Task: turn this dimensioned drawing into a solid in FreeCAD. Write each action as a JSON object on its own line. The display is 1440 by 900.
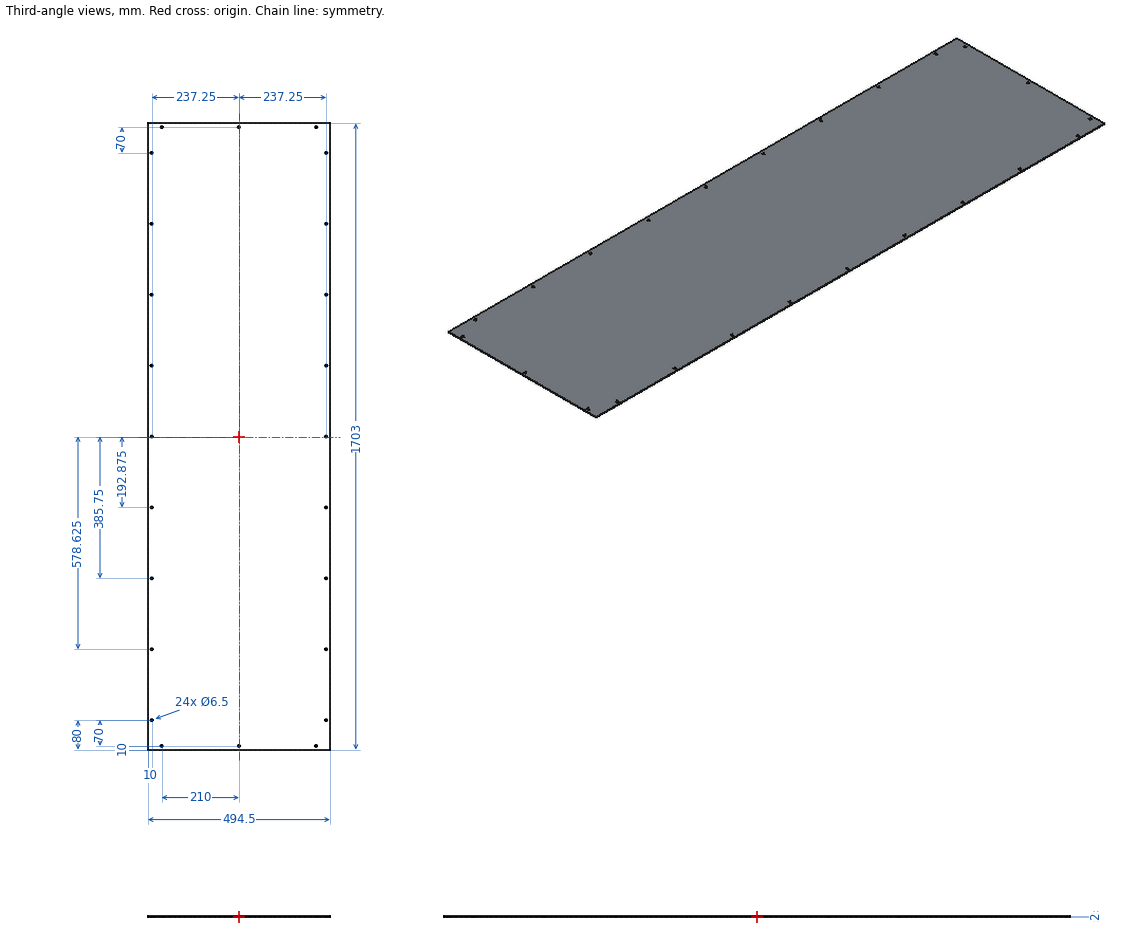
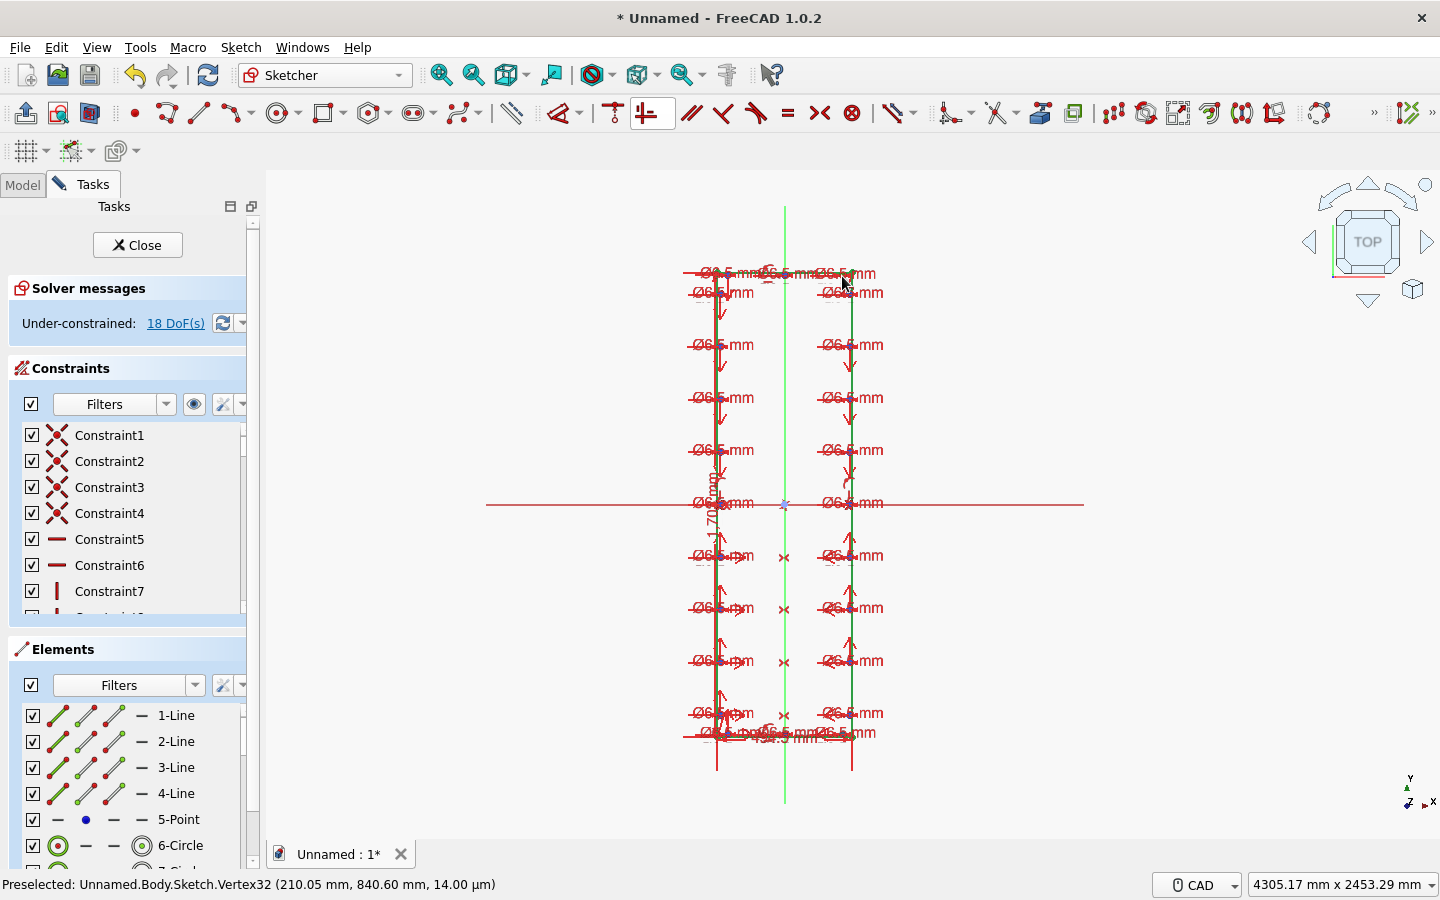
{"action": "left_click", "coordinate": [504, 505]}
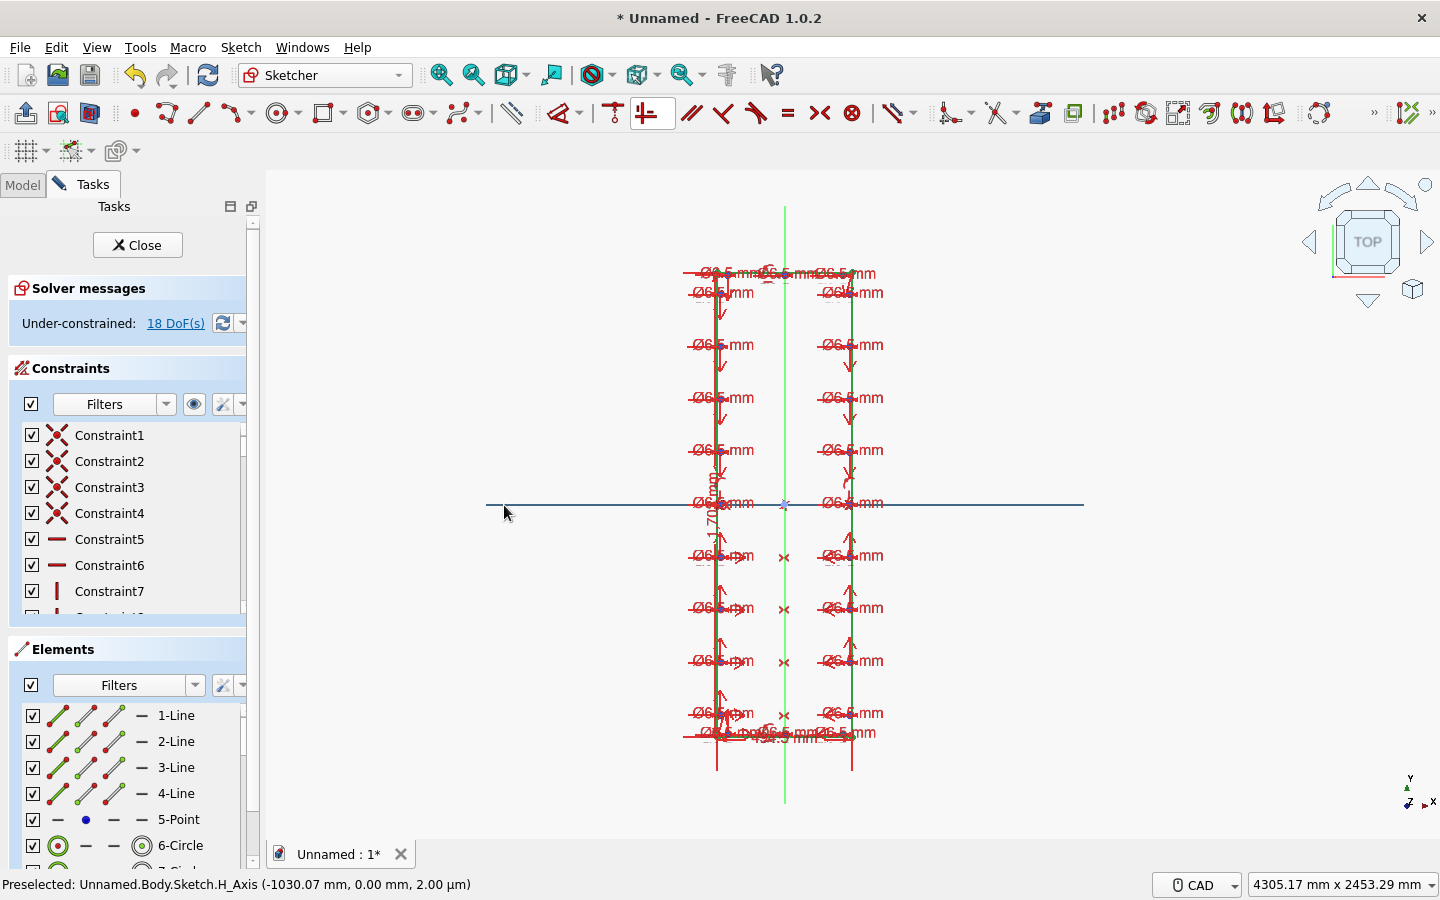
{"action": "left_click", "coordinate": [820, 114]}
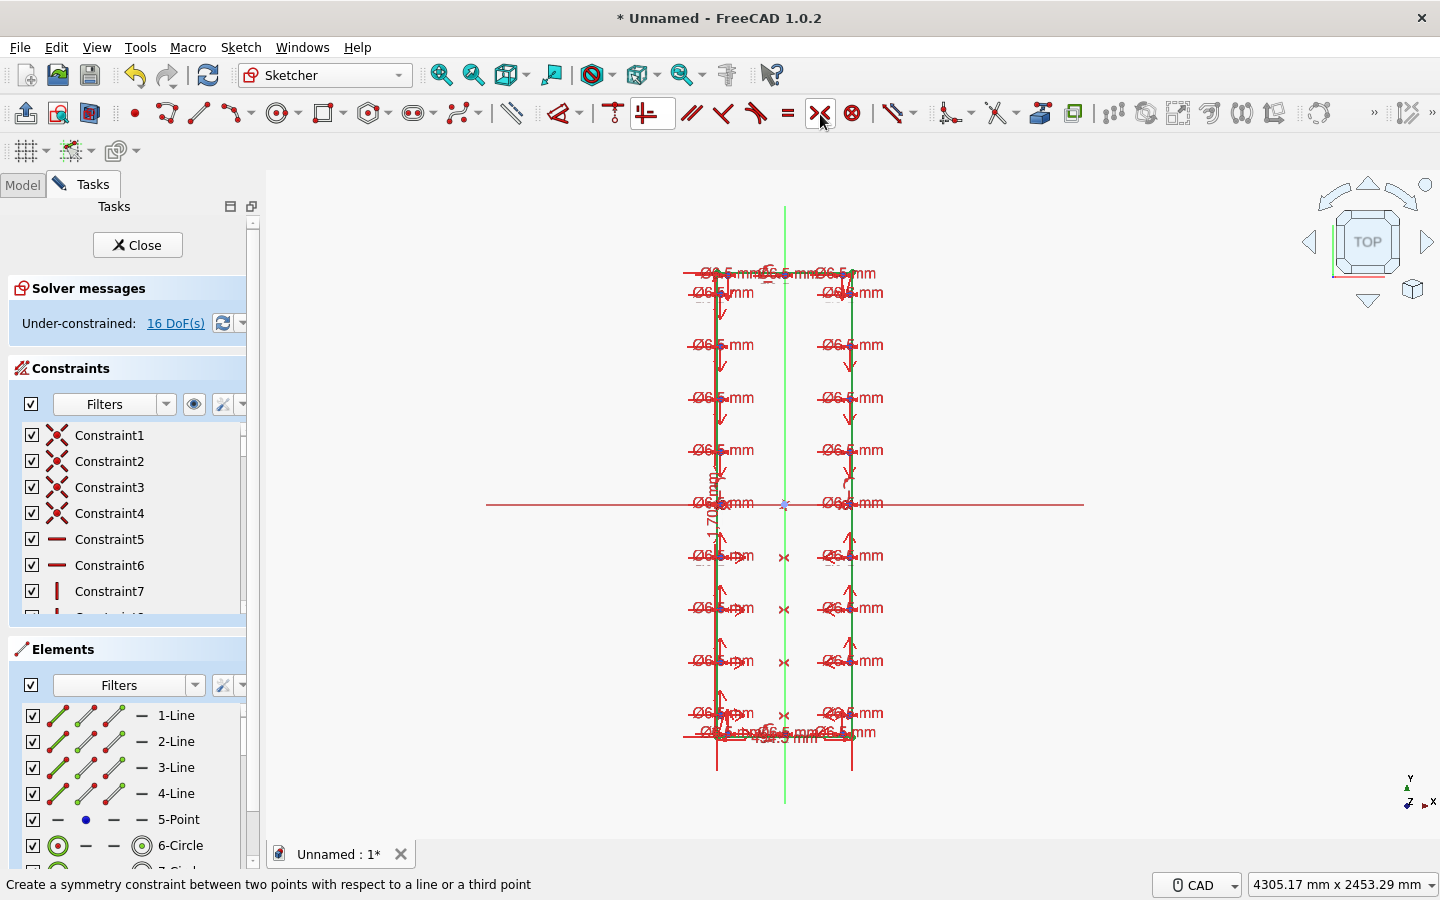
{"action": "left_click", "coordinate": [850, 715]}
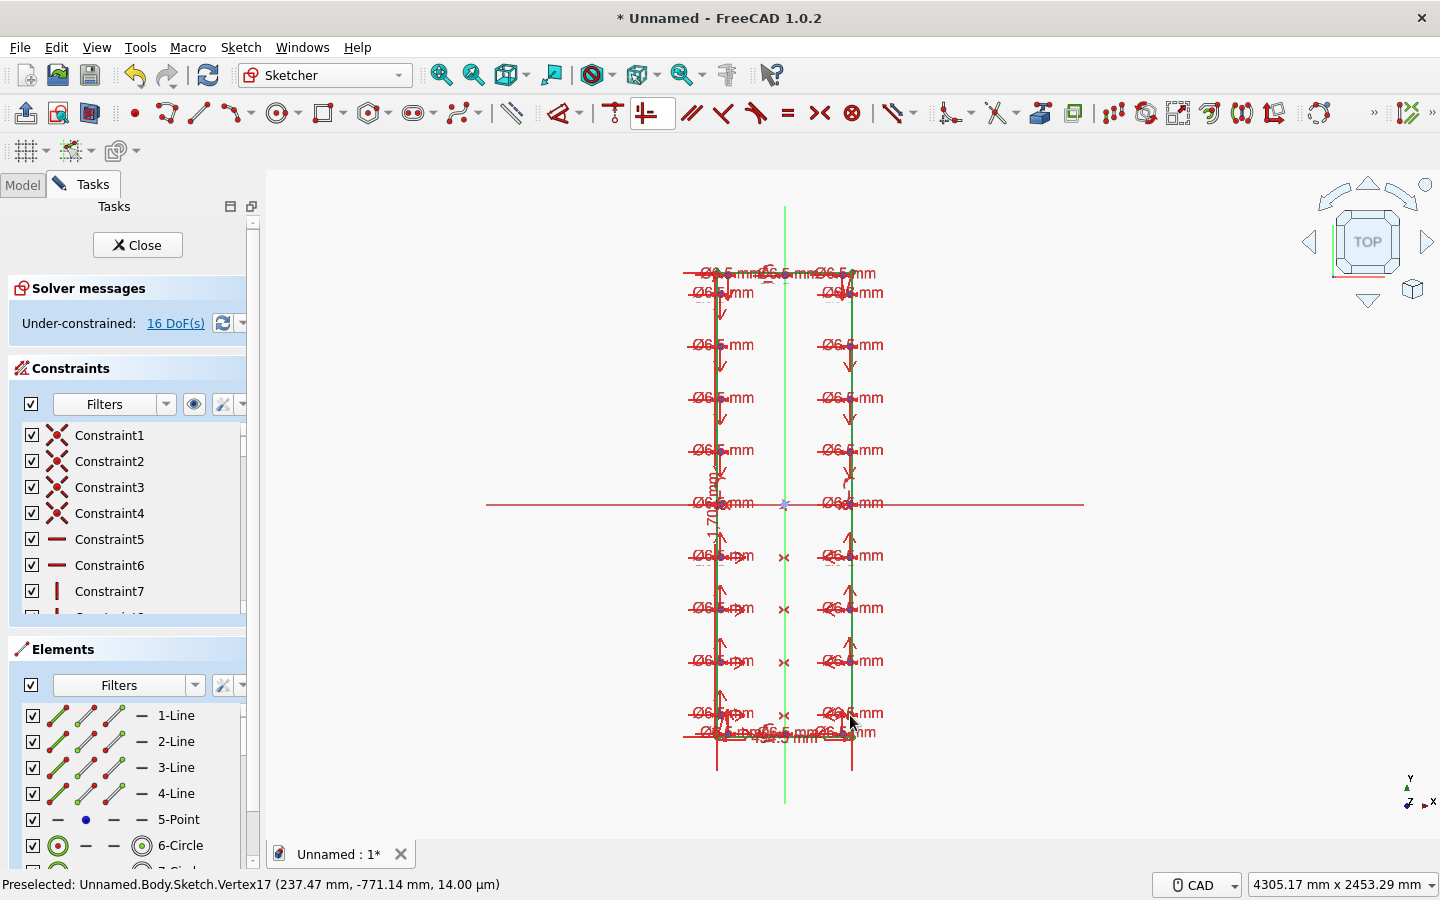
{"action": "left_click", "coordinate": [850, 295]}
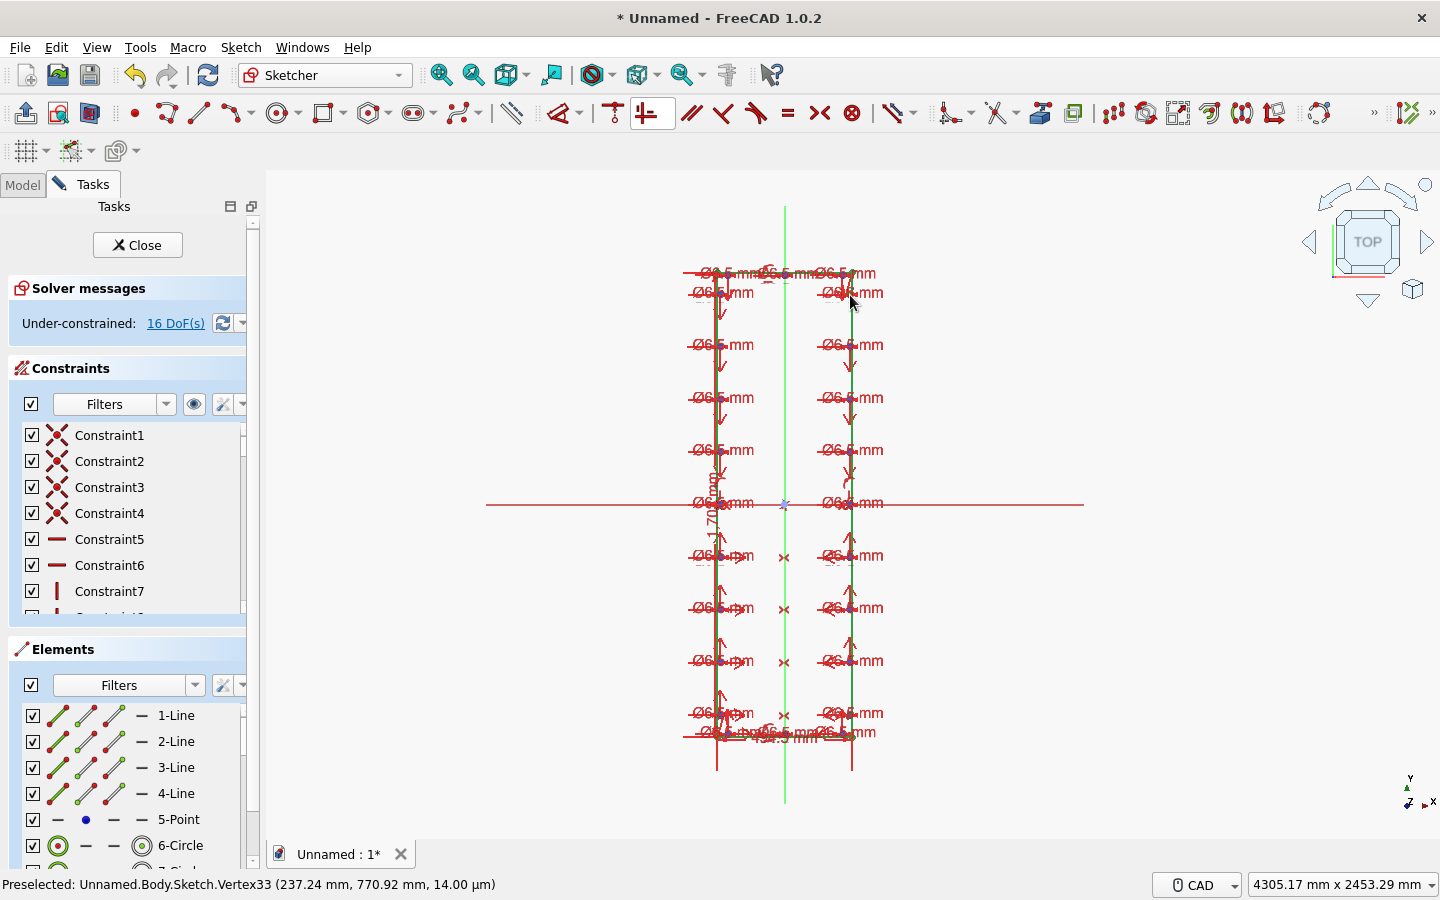
{"action": "left_click", "coordinate": [504, 505]}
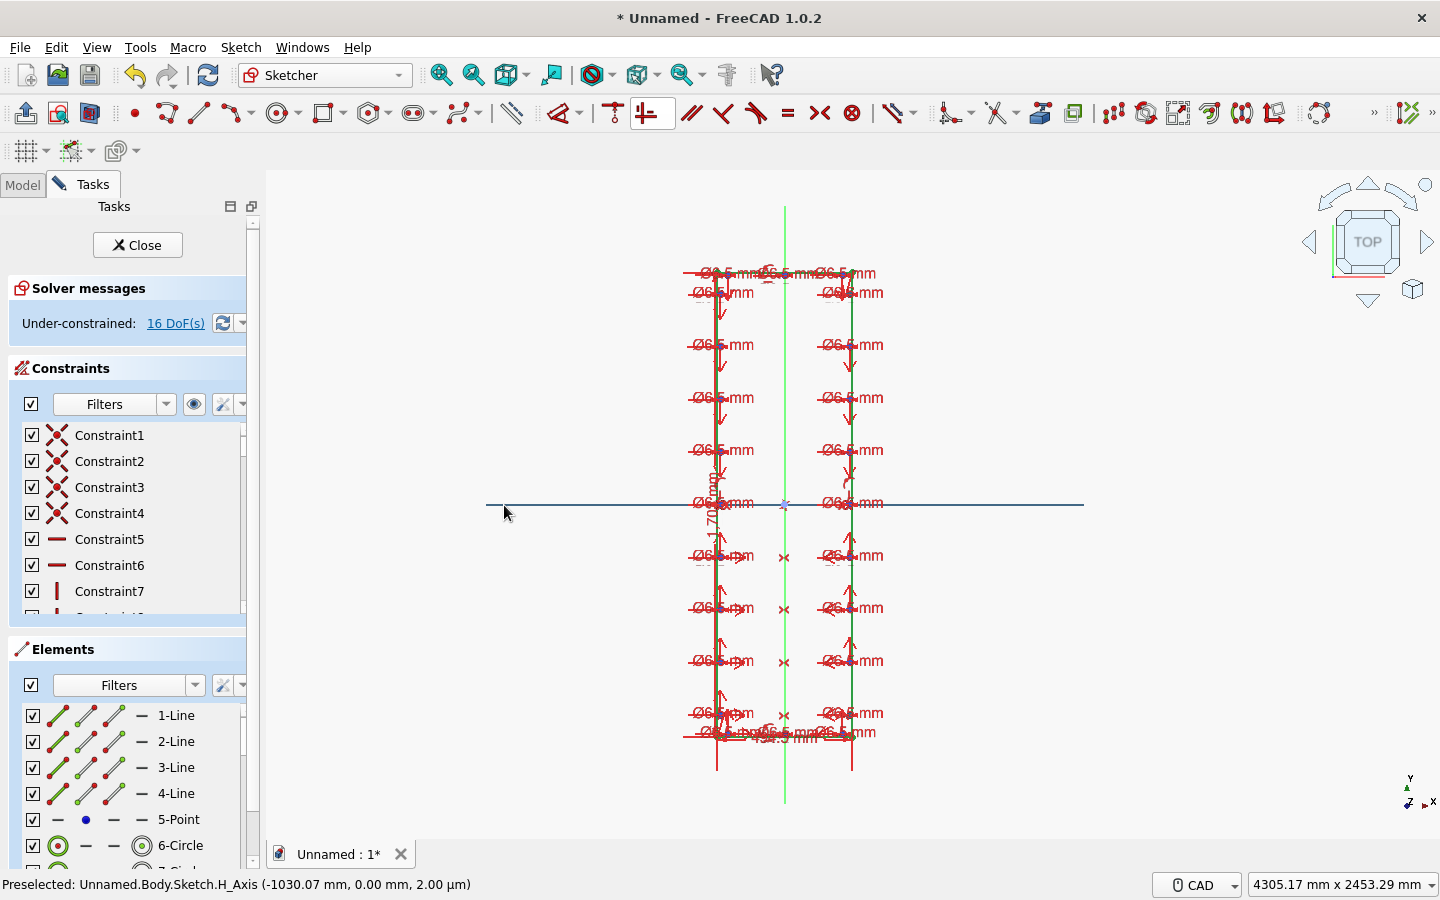
{"action": "left_click", "coordinate": [820, 114]}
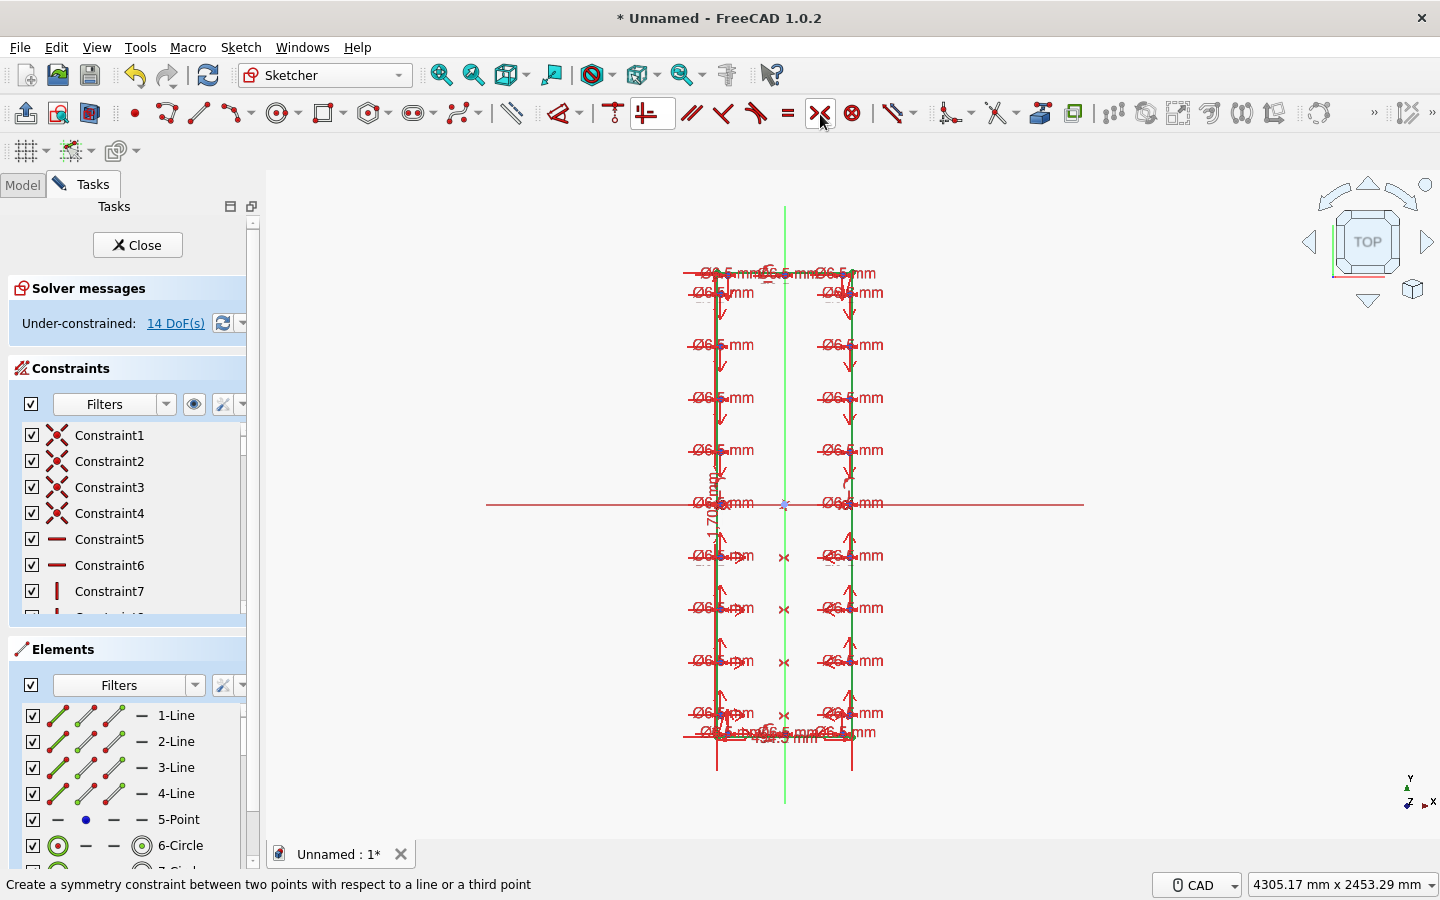
{"action": "left_click", "coordinate": [558, 114]}